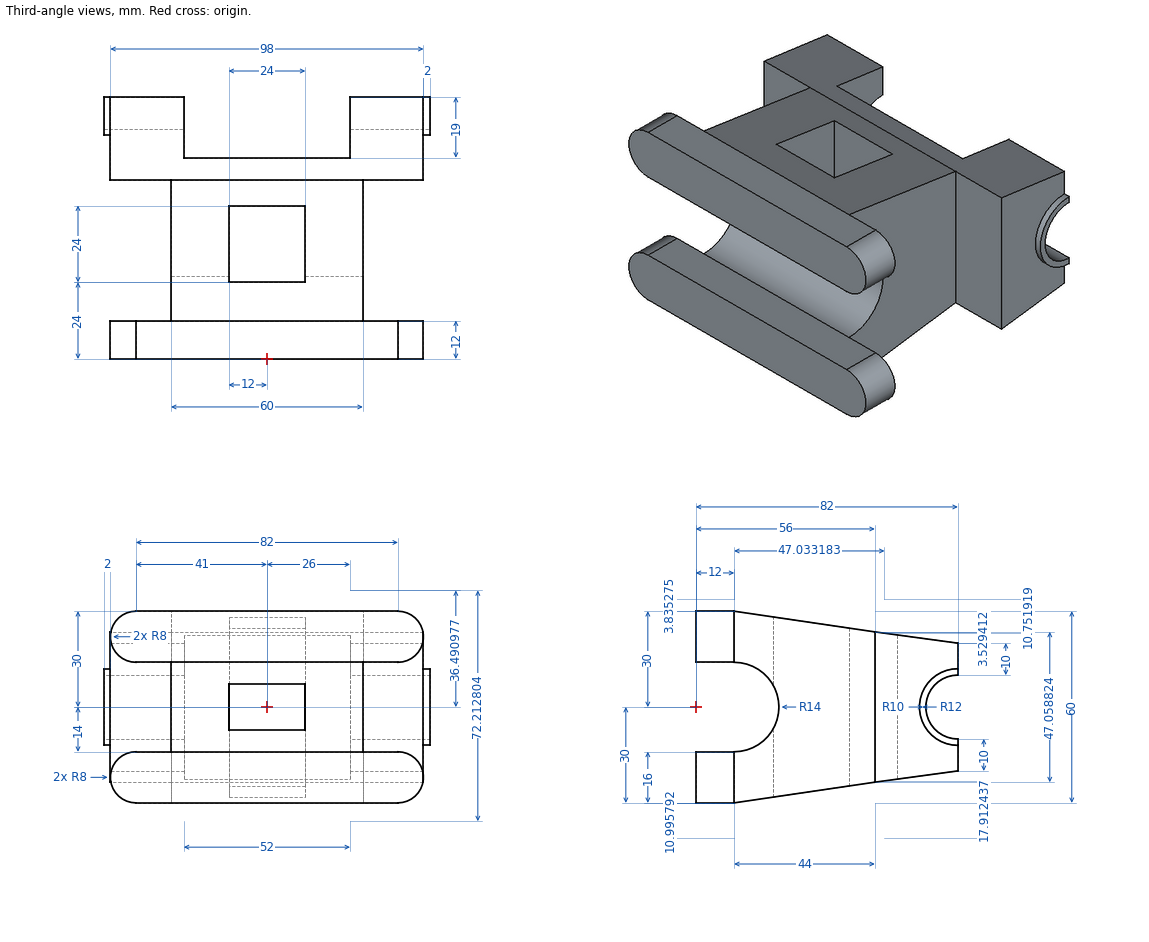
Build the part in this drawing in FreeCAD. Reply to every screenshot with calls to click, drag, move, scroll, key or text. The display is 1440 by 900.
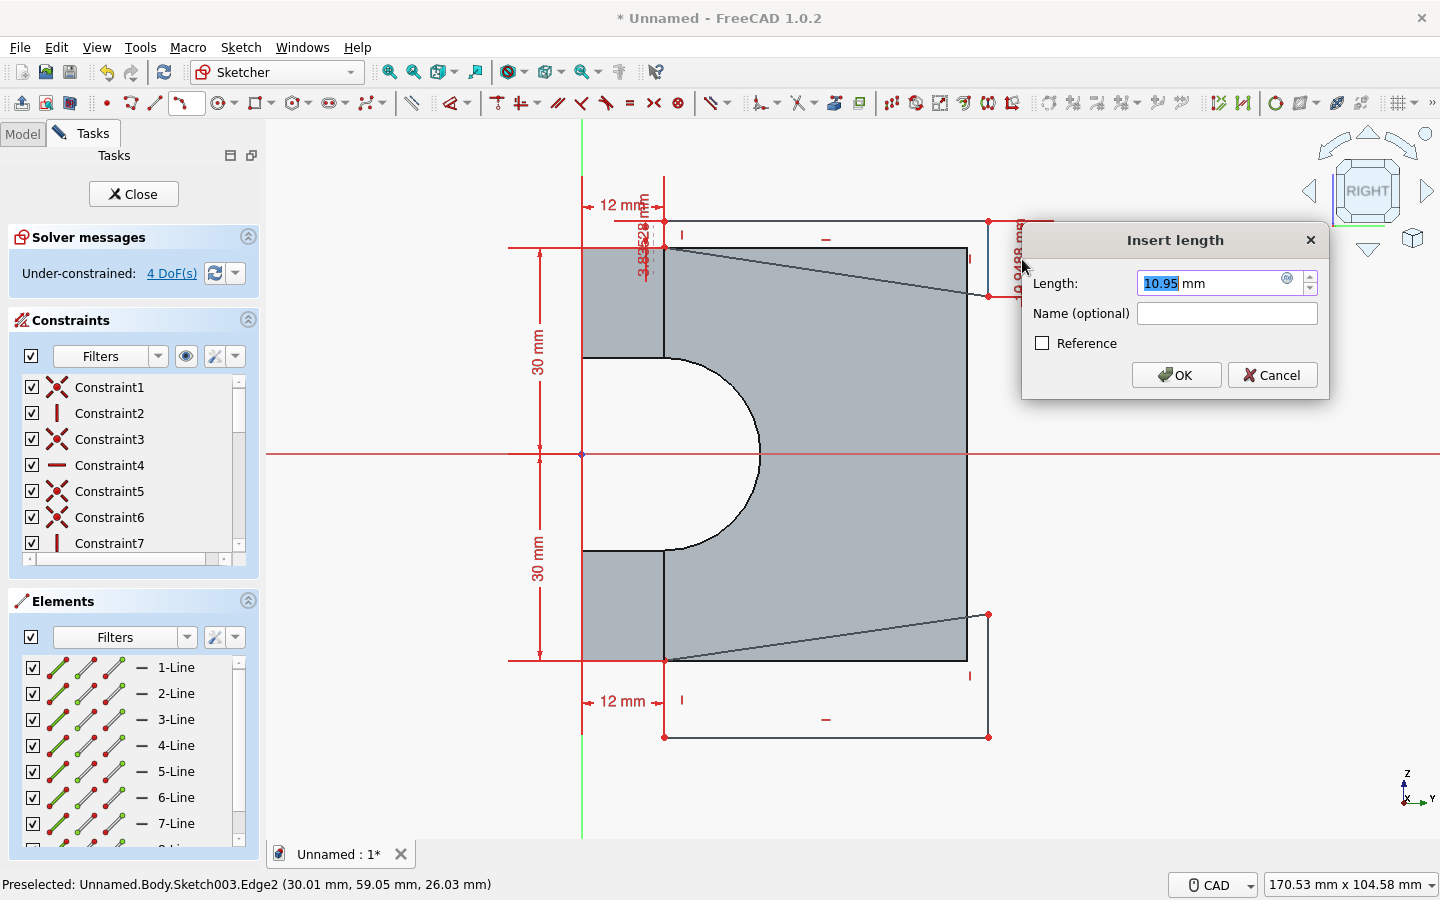
text(10.751919)
key(Return)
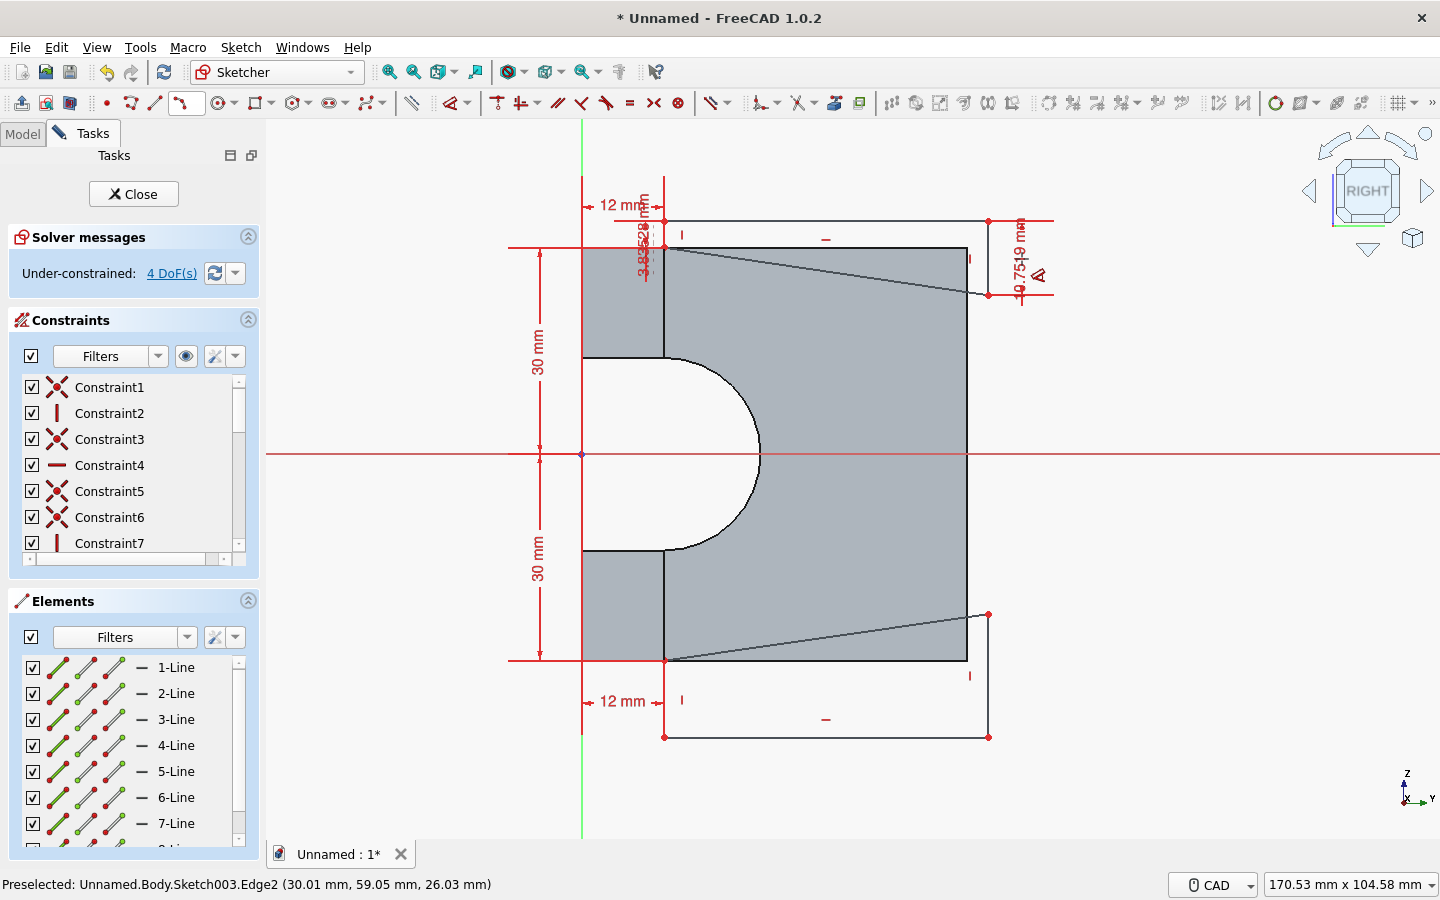
click(891, 221)
click(826, 187)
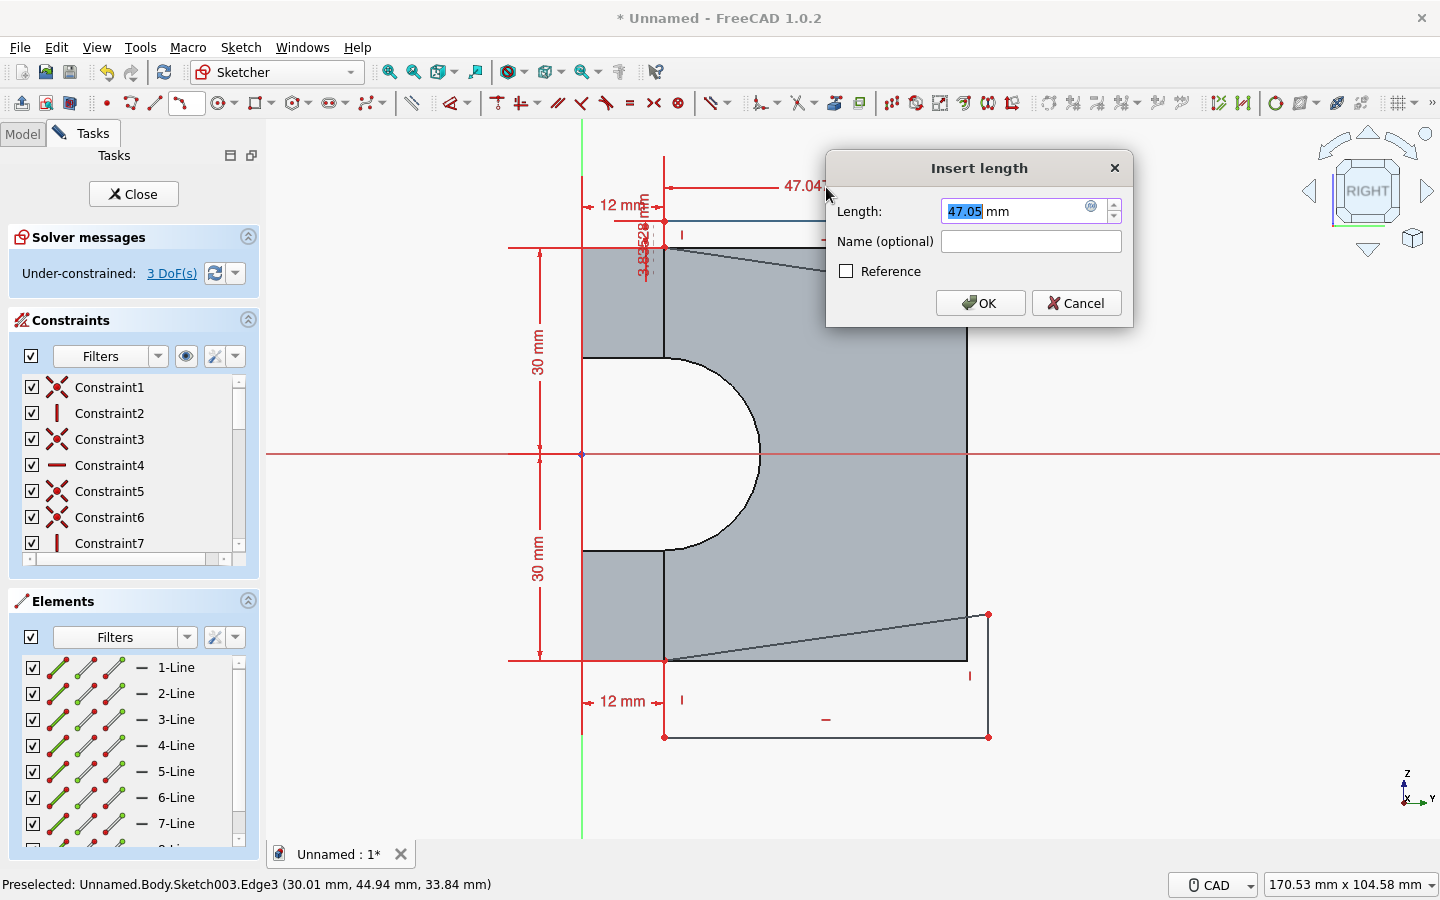
text(47.033183)
key(Return)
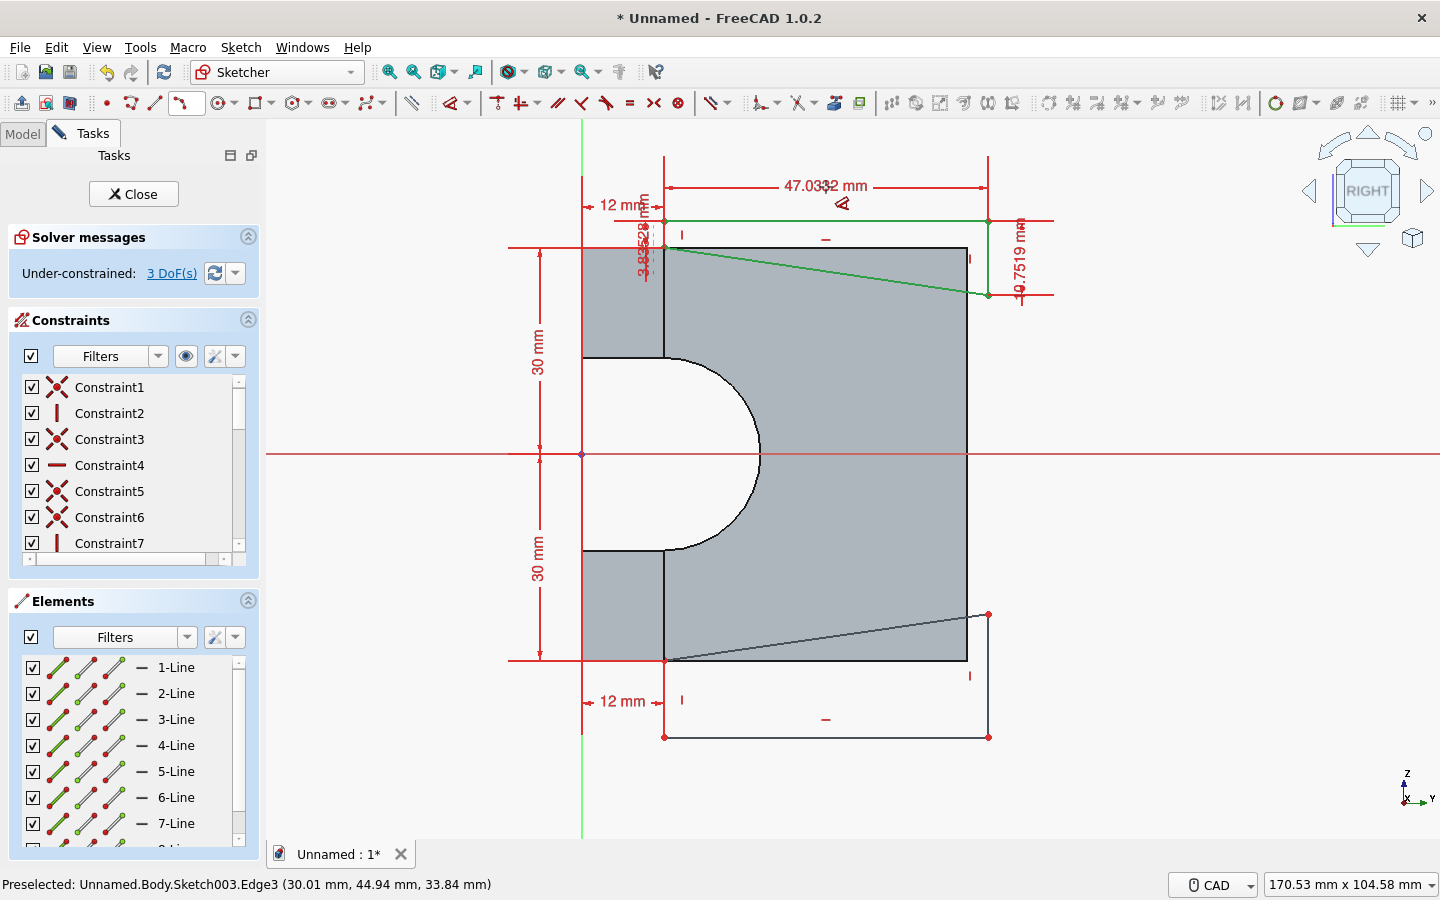
click(664, 684)
click(630, 681)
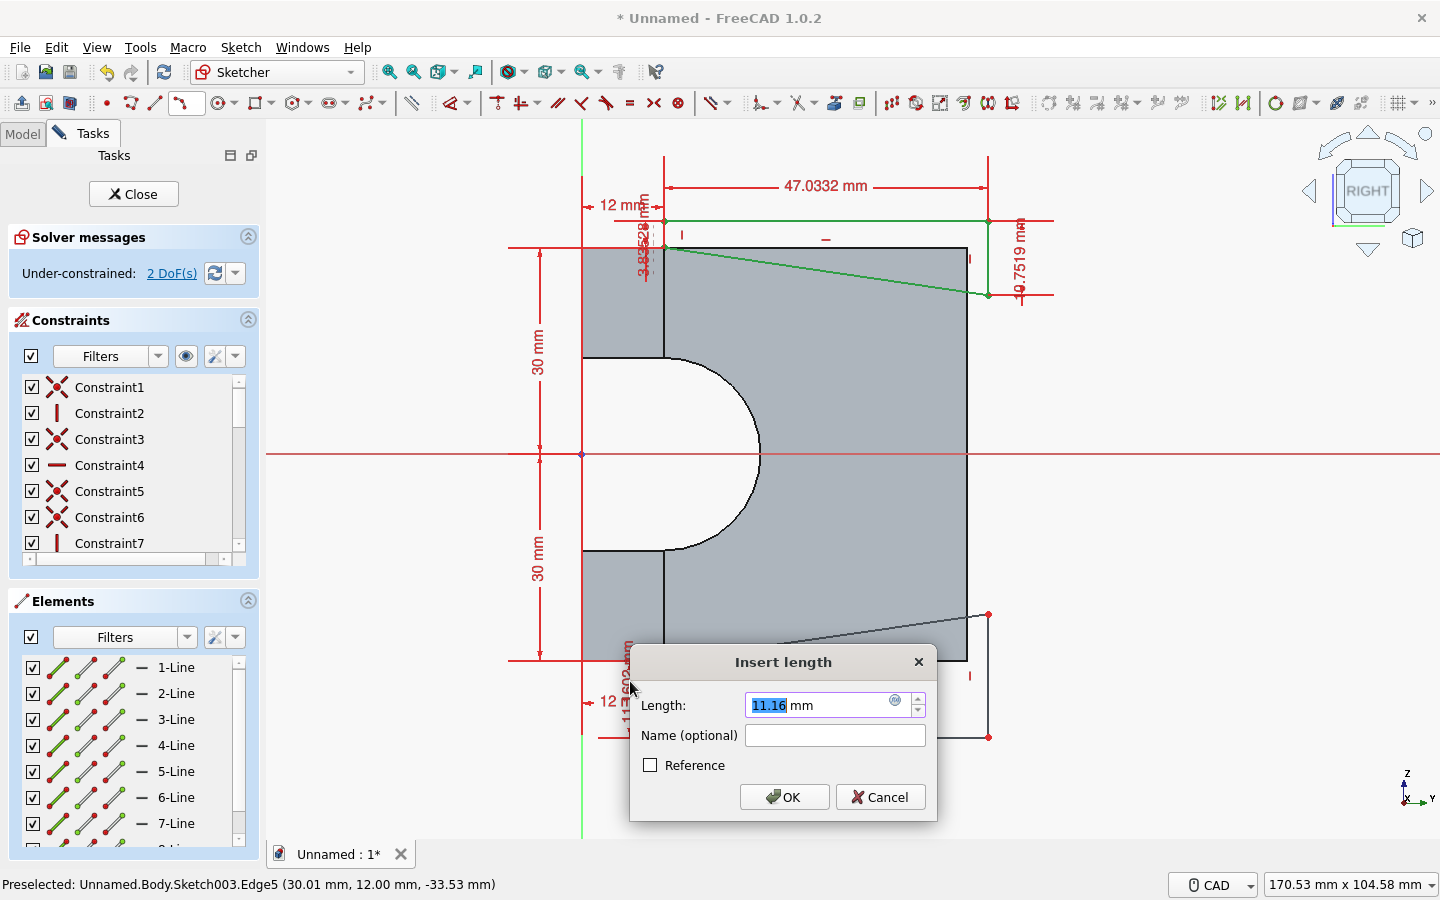
text(10.995792)
key(Return)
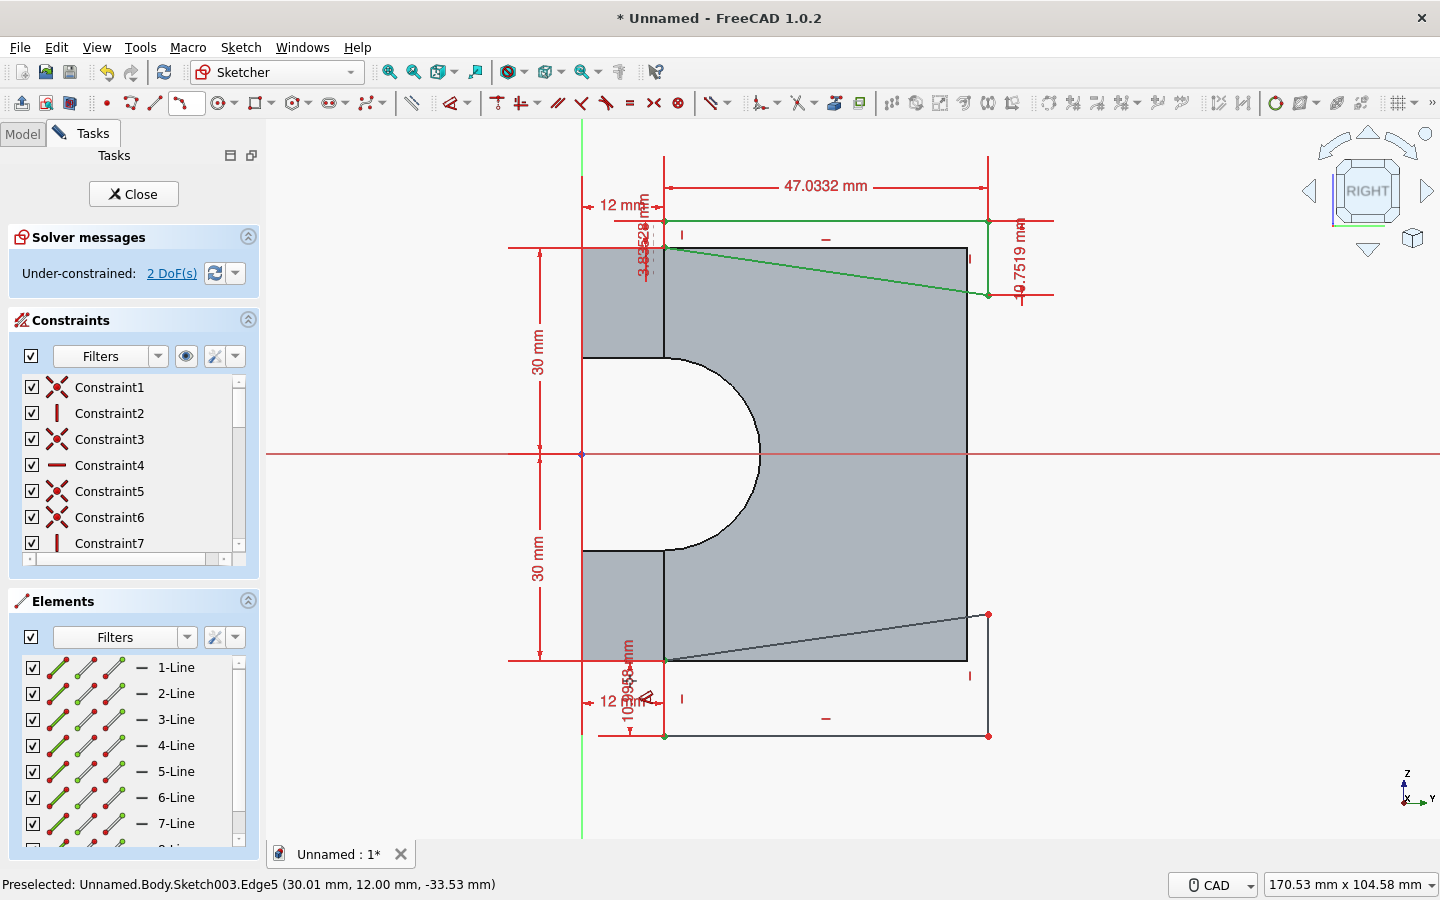
click(761, 736)
click(826, 770)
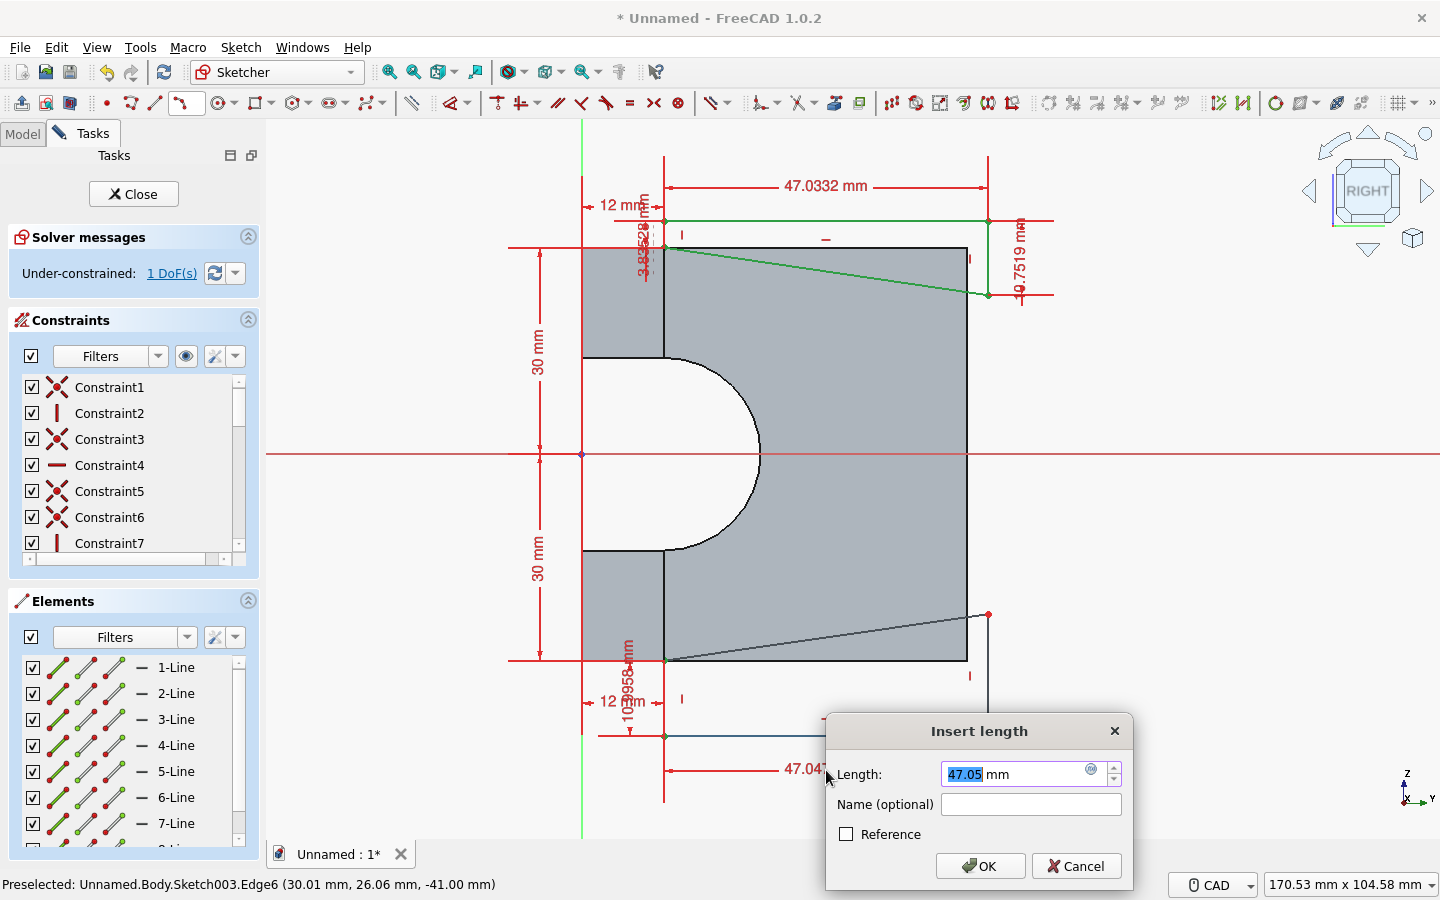
text(47.033183)
key(Return)